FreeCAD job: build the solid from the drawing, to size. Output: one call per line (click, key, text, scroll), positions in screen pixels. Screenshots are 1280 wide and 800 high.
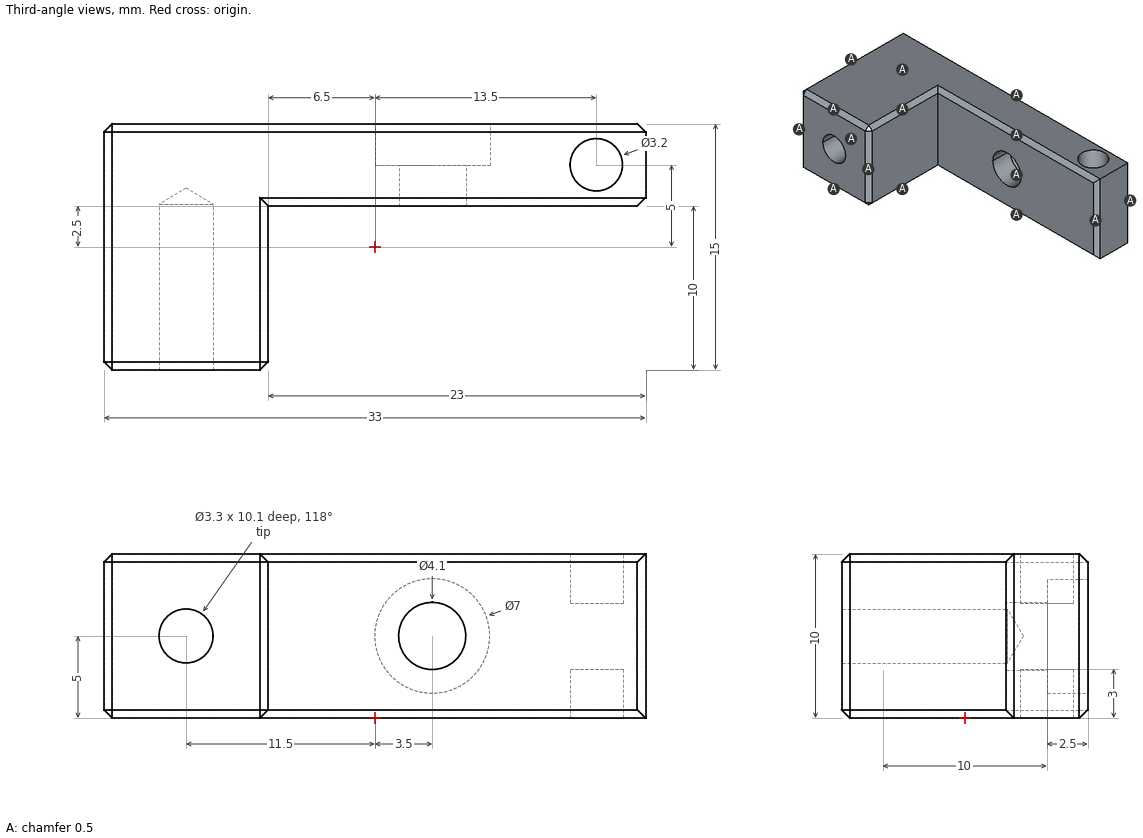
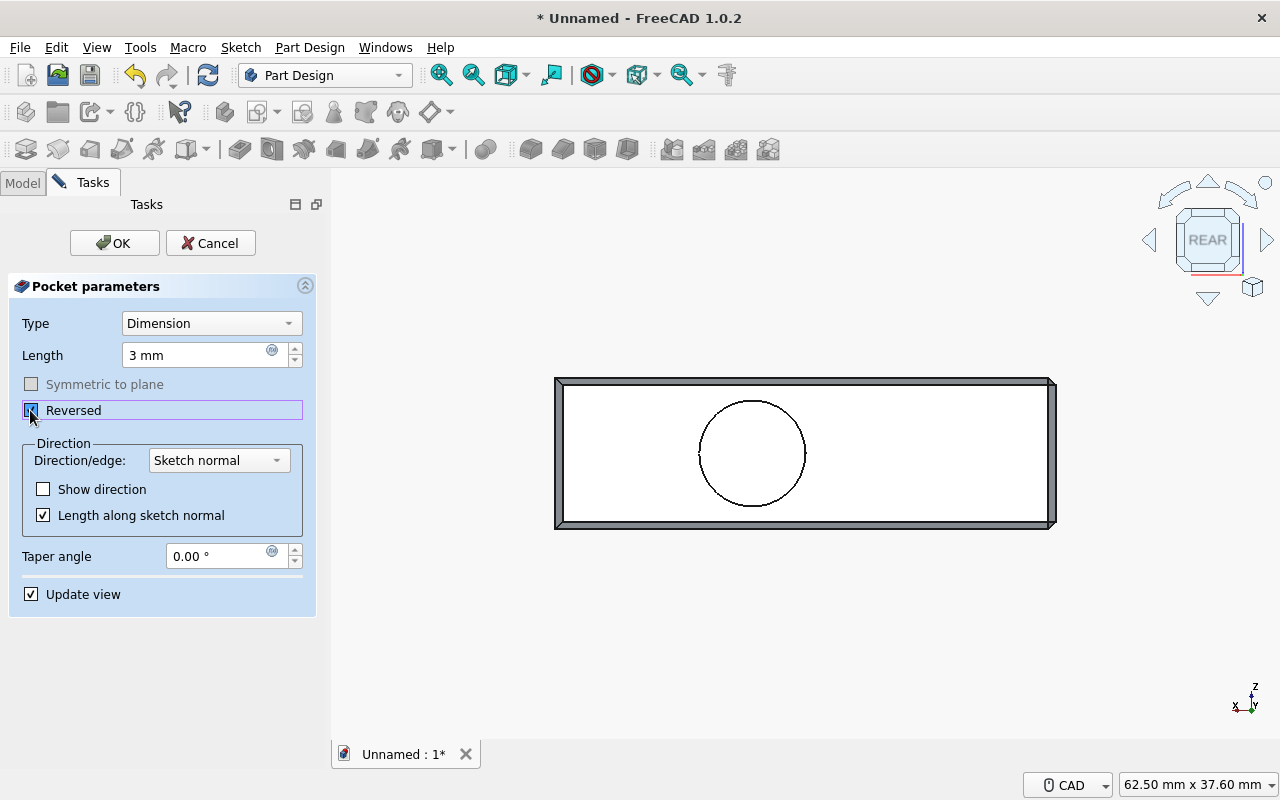
click(115, 243)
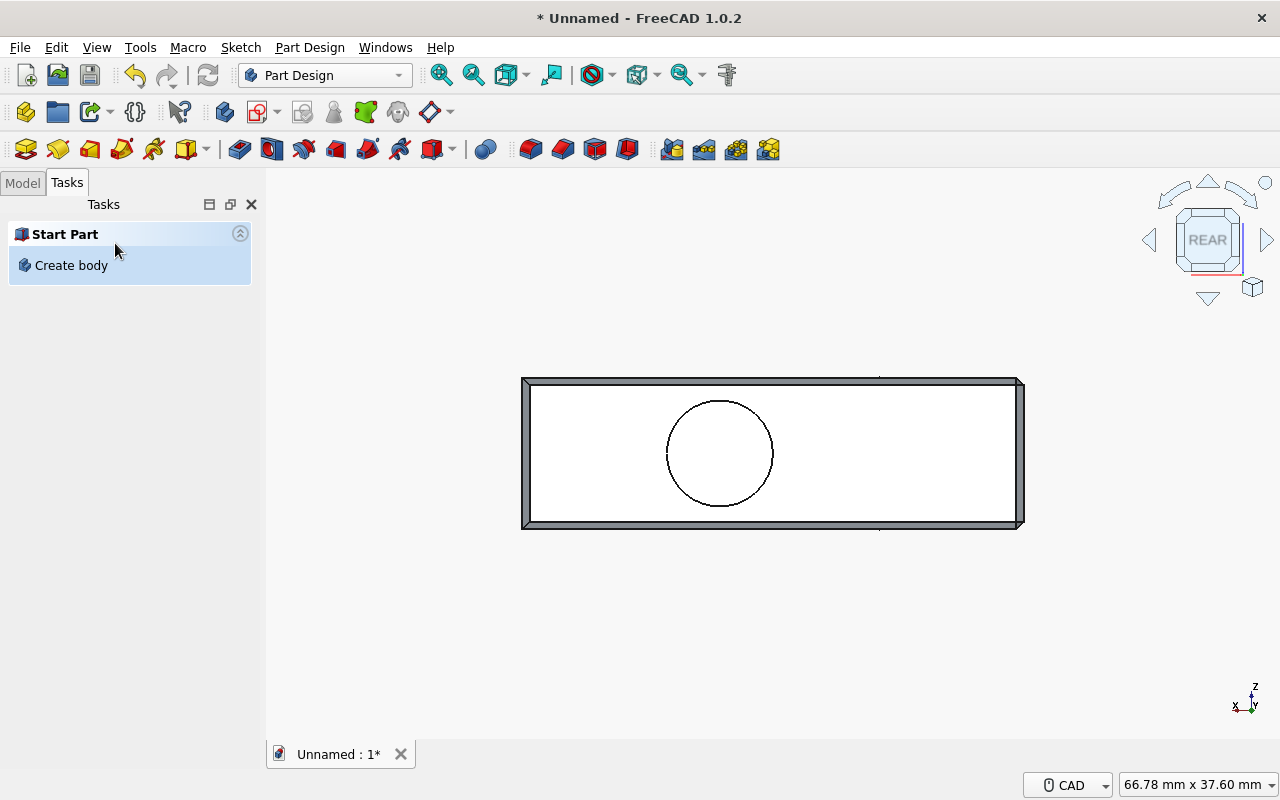
click(23, 182)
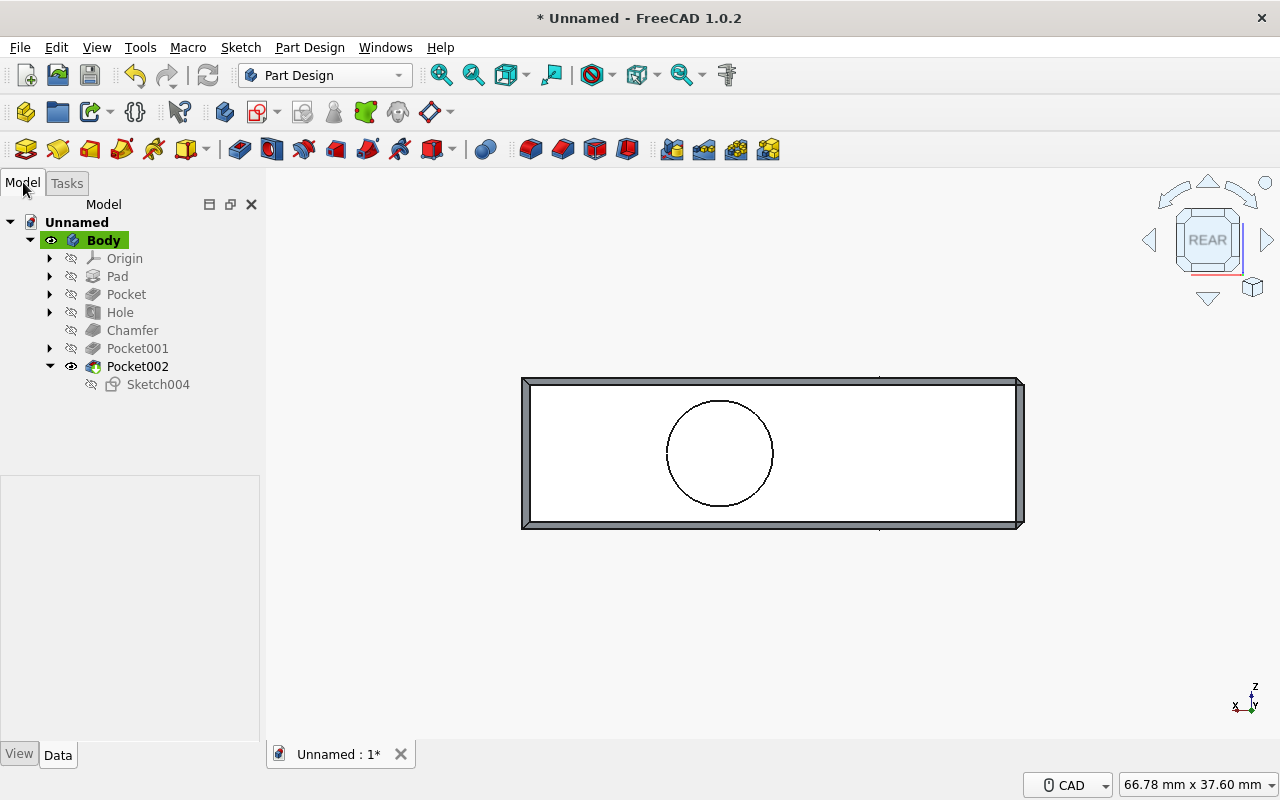
click(50, 258)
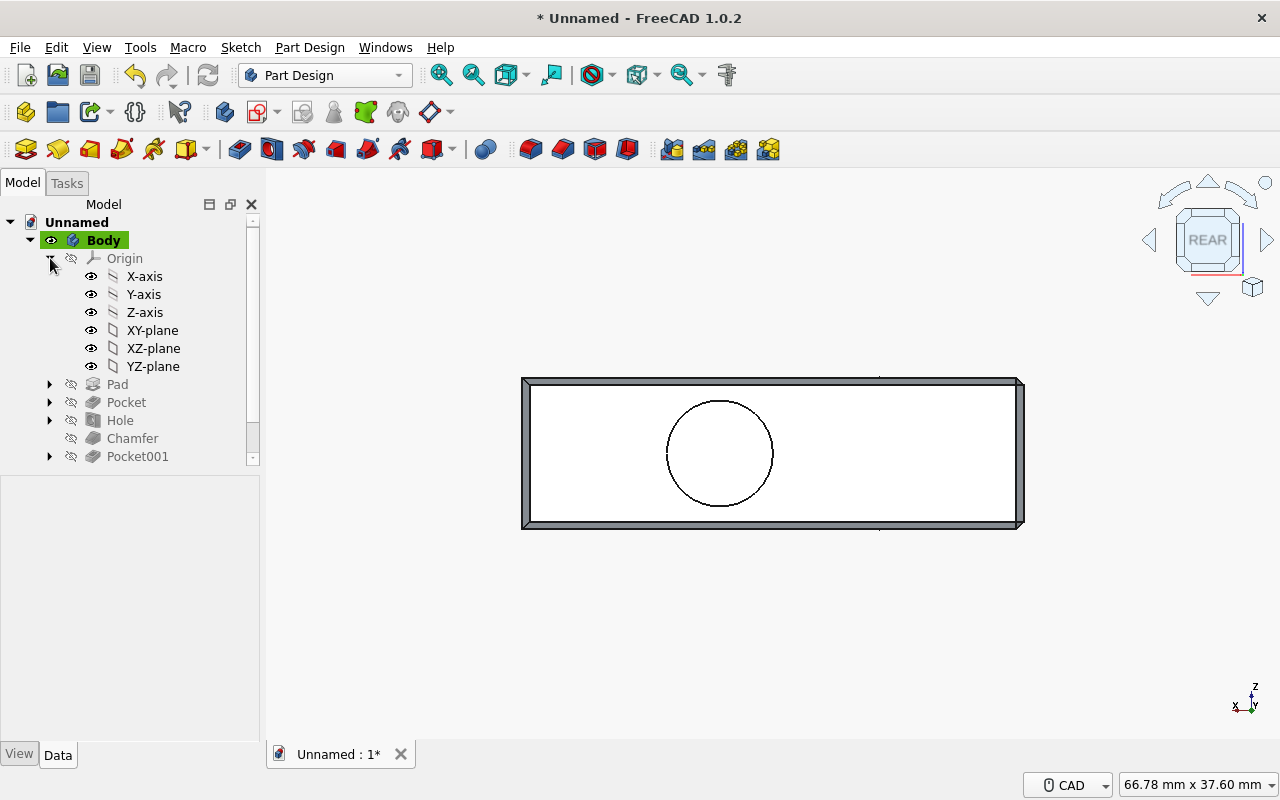
click(136, 330)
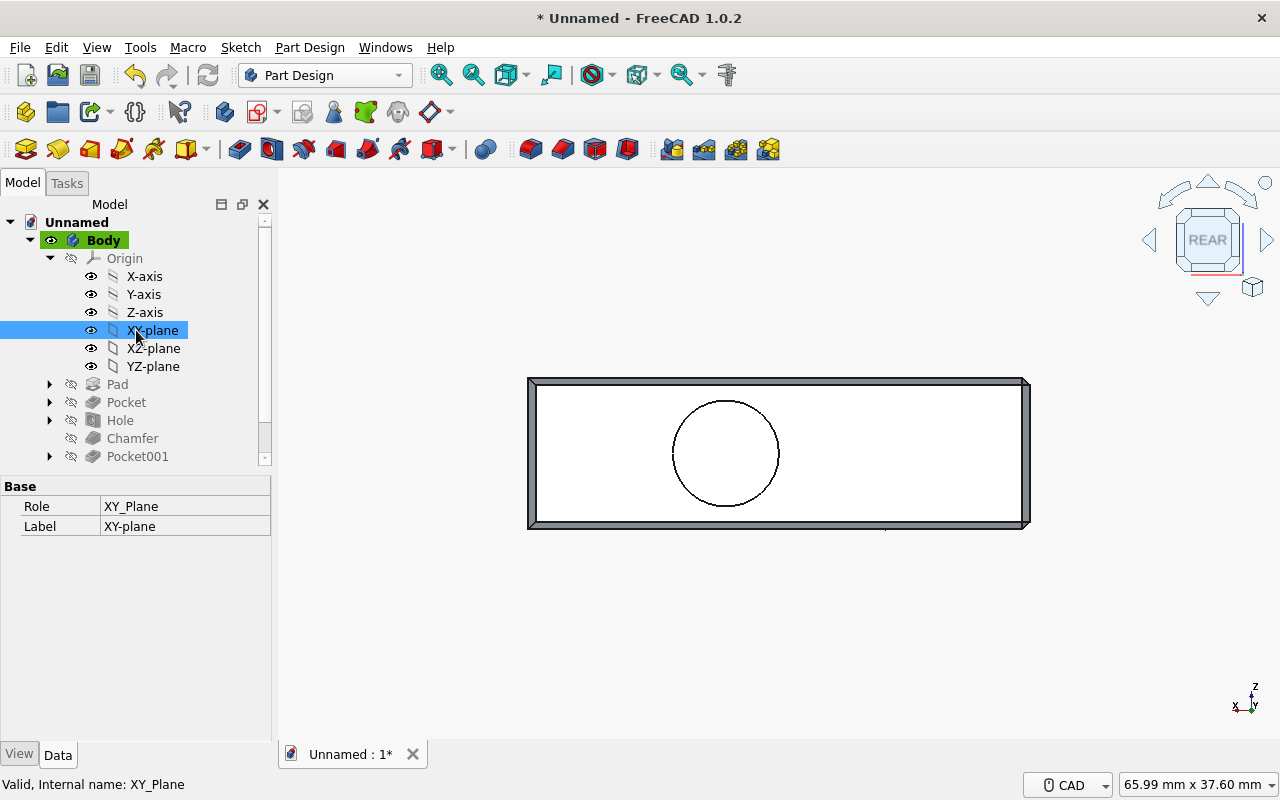
click(430, 112)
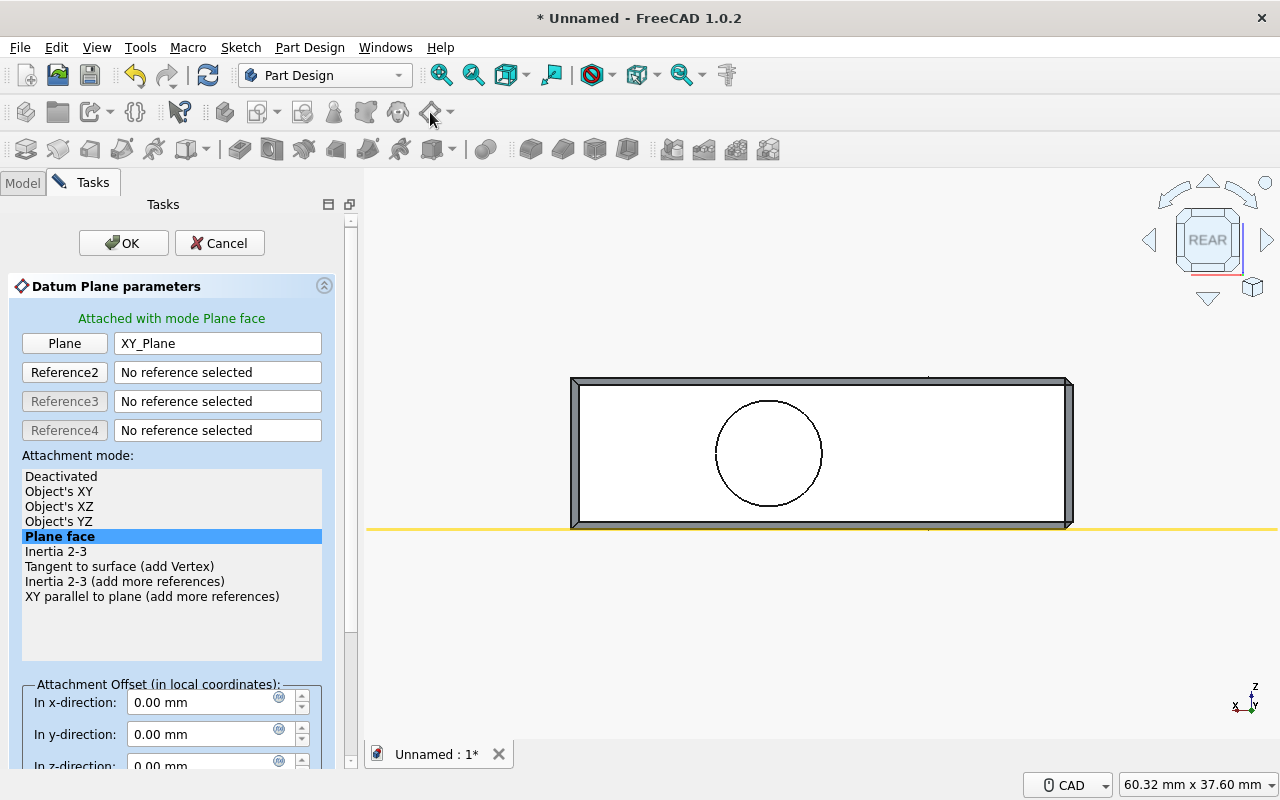
scroll(351, 491, down, 2)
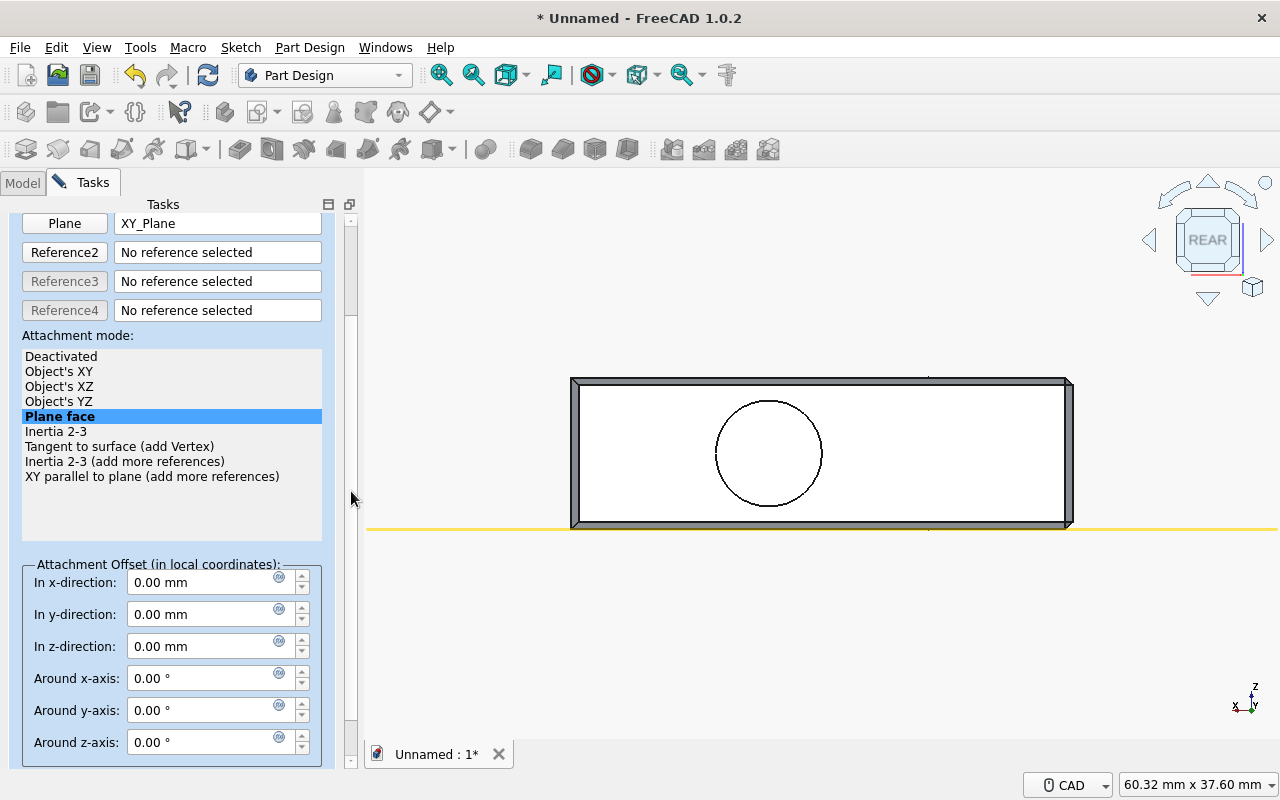
triple_click(210, 646)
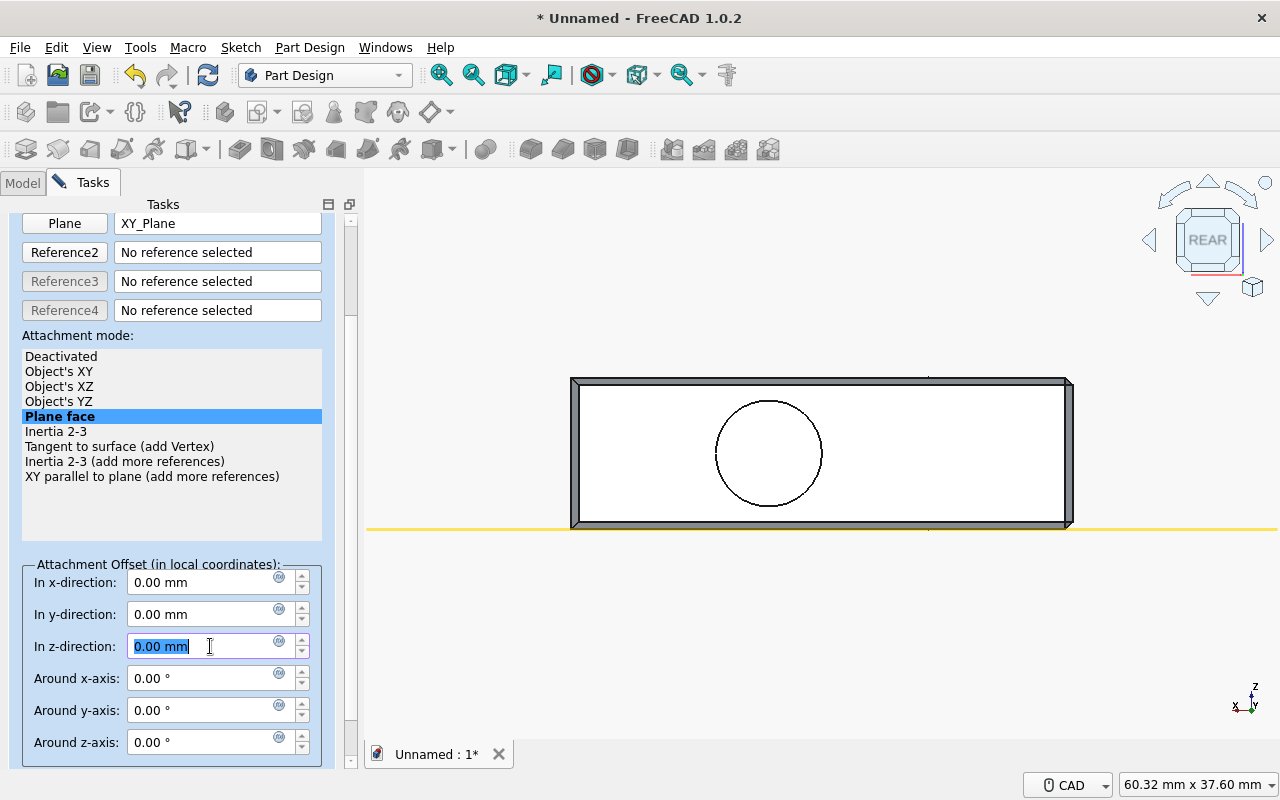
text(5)
key(Tab)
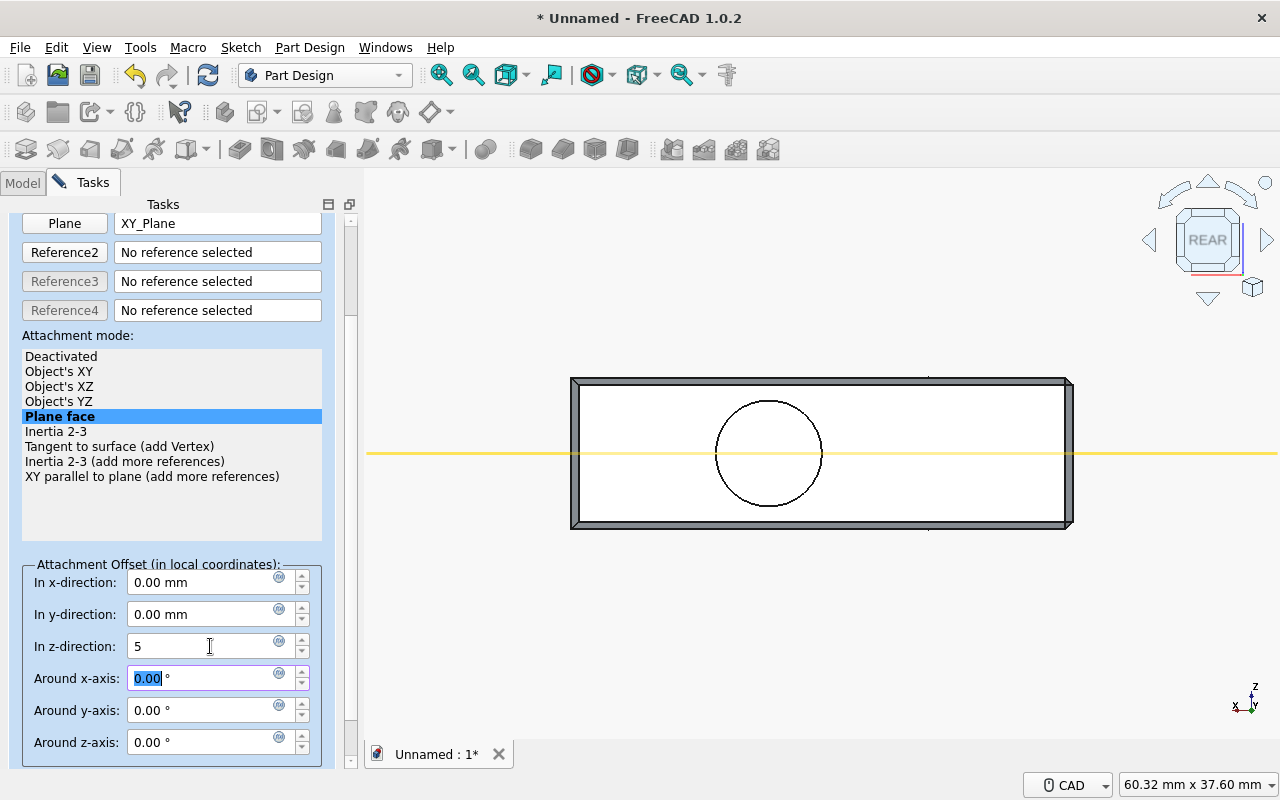
scroll(351, 491, up, 3)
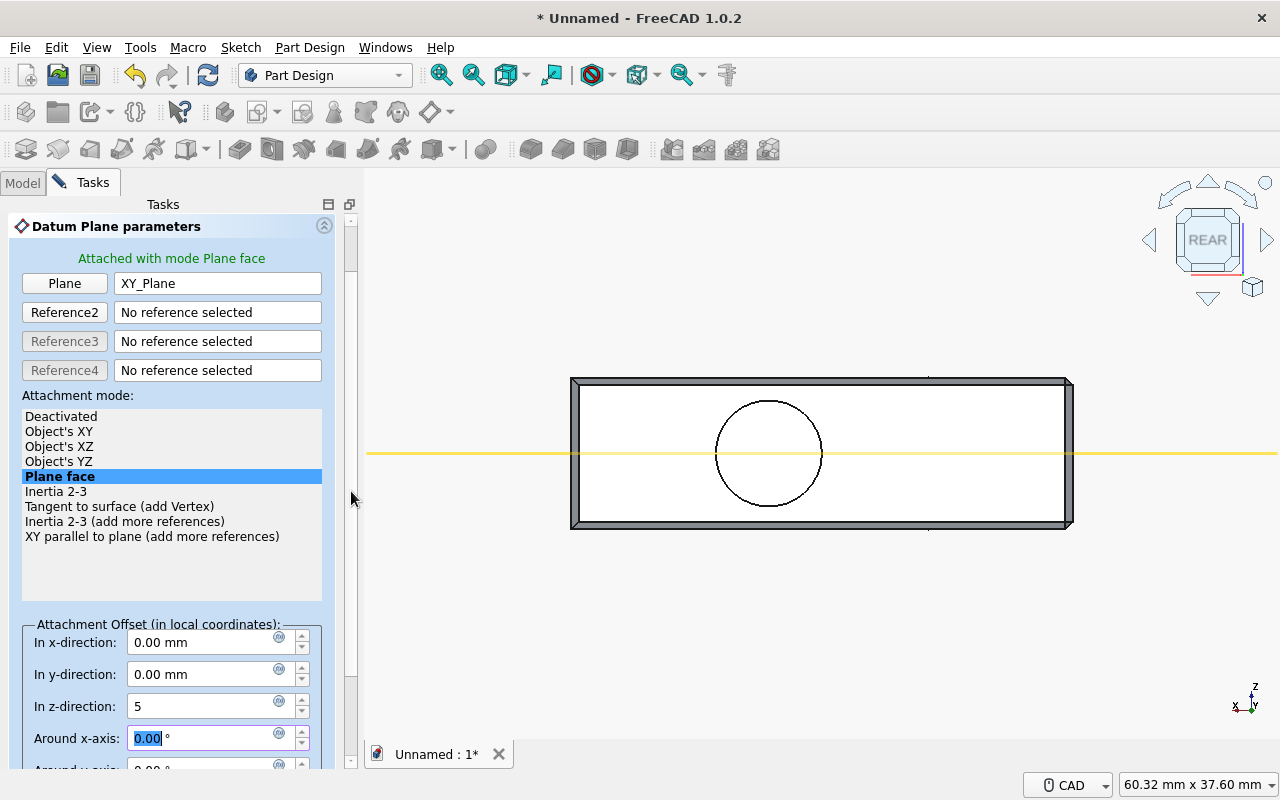
click(124, 243)